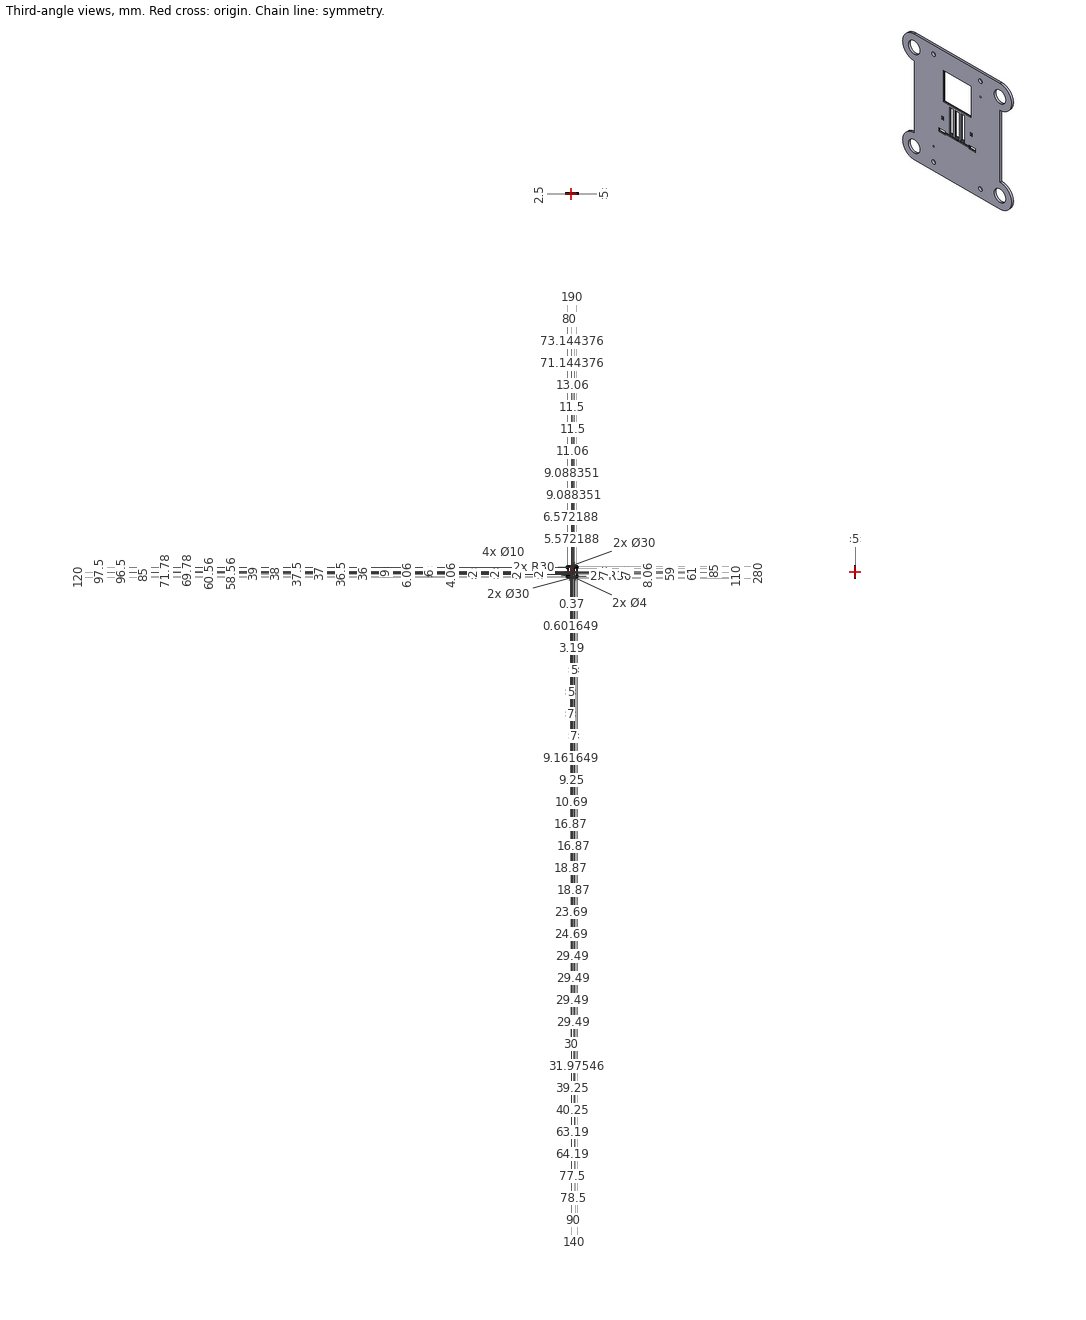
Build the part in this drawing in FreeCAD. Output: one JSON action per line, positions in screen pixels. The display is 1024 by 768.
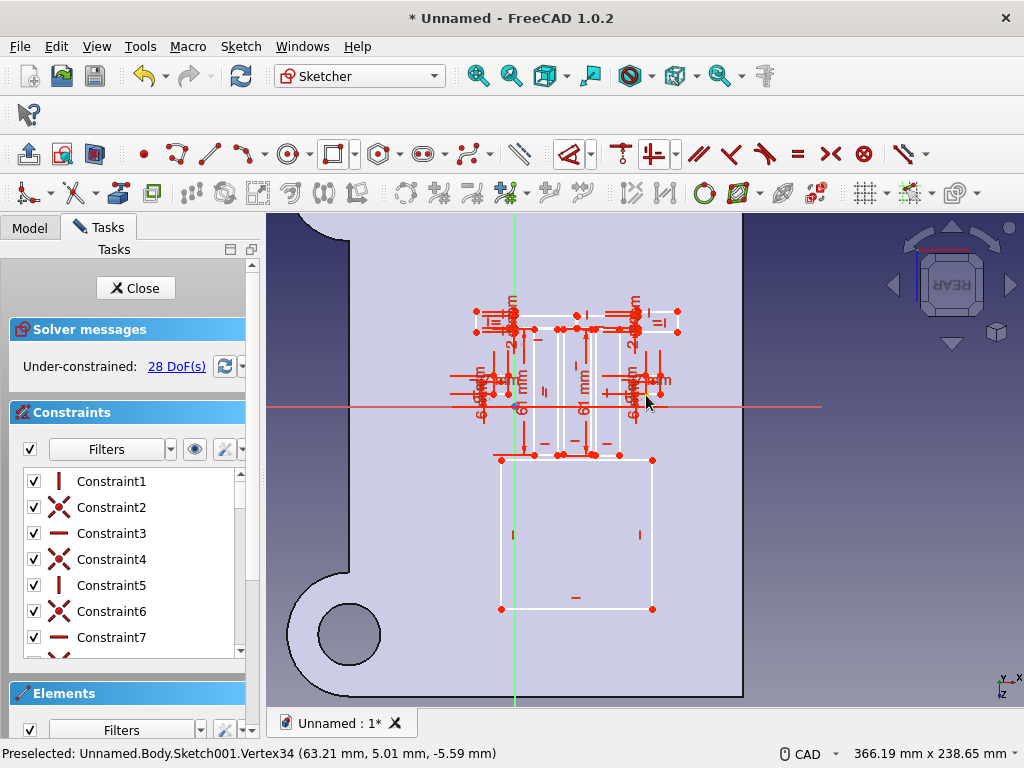
{"action": "scroll", "coordinate": [516, 332], "scroll_direction": "up", "scroll_amount": 6}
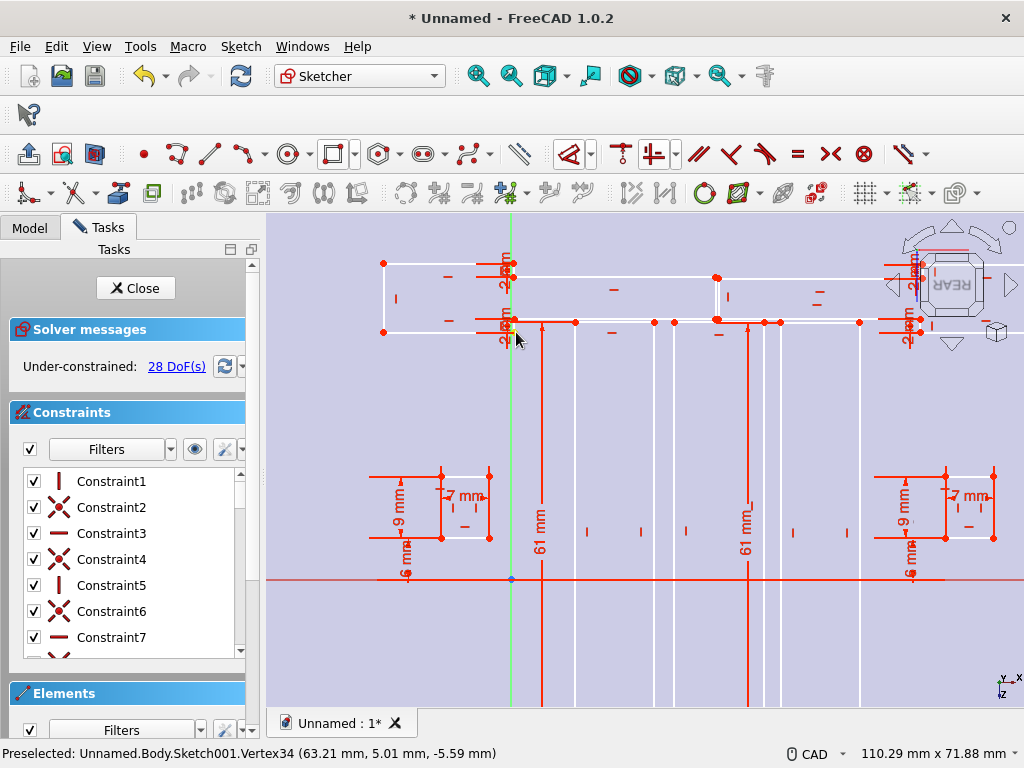
{"action": "left_click", "coordinate": [514, 333]}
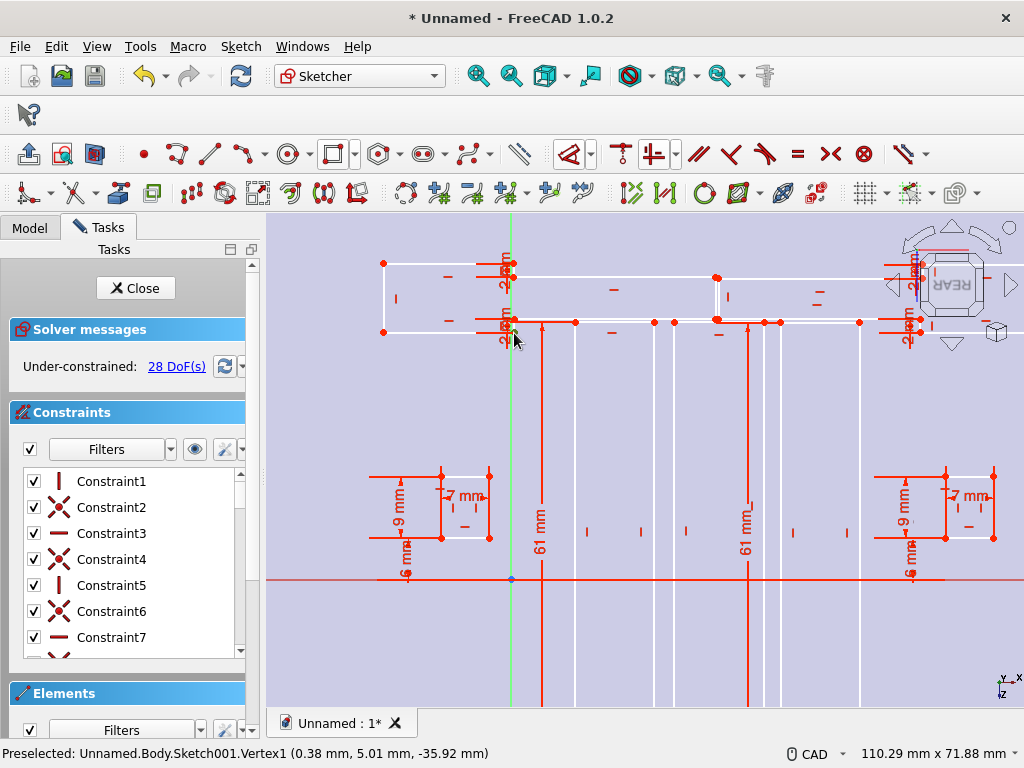
{"action": "left_click", "coordinate": [590, 154]}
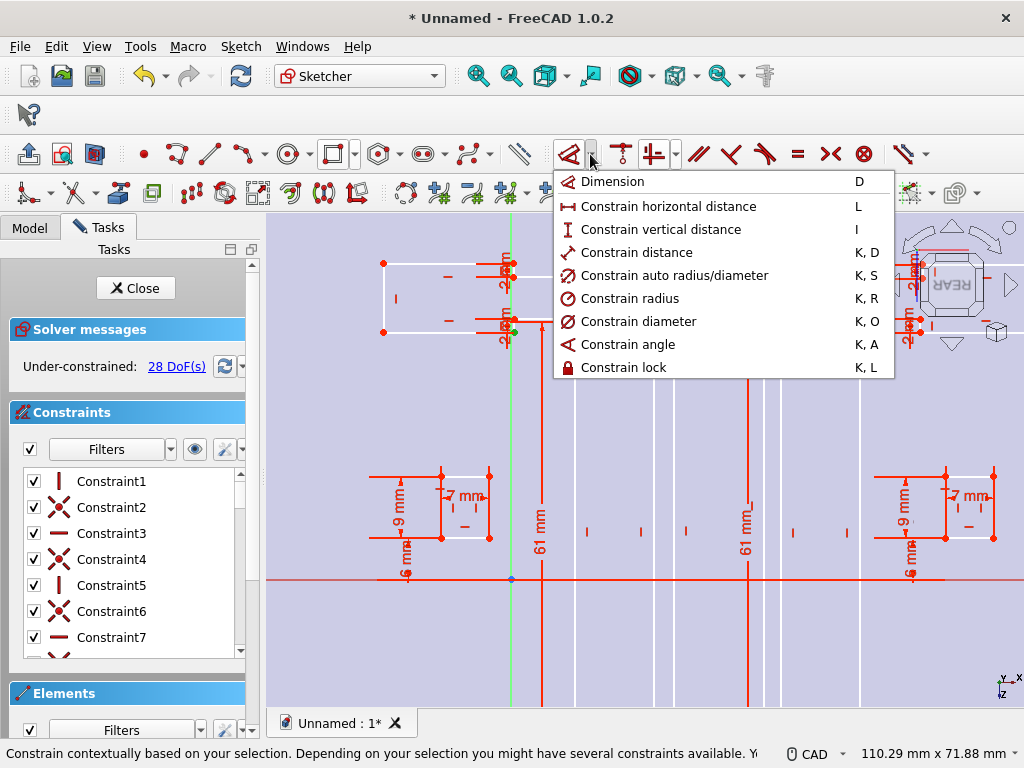
{"action": "left_click", "coordinate": [724, 230]}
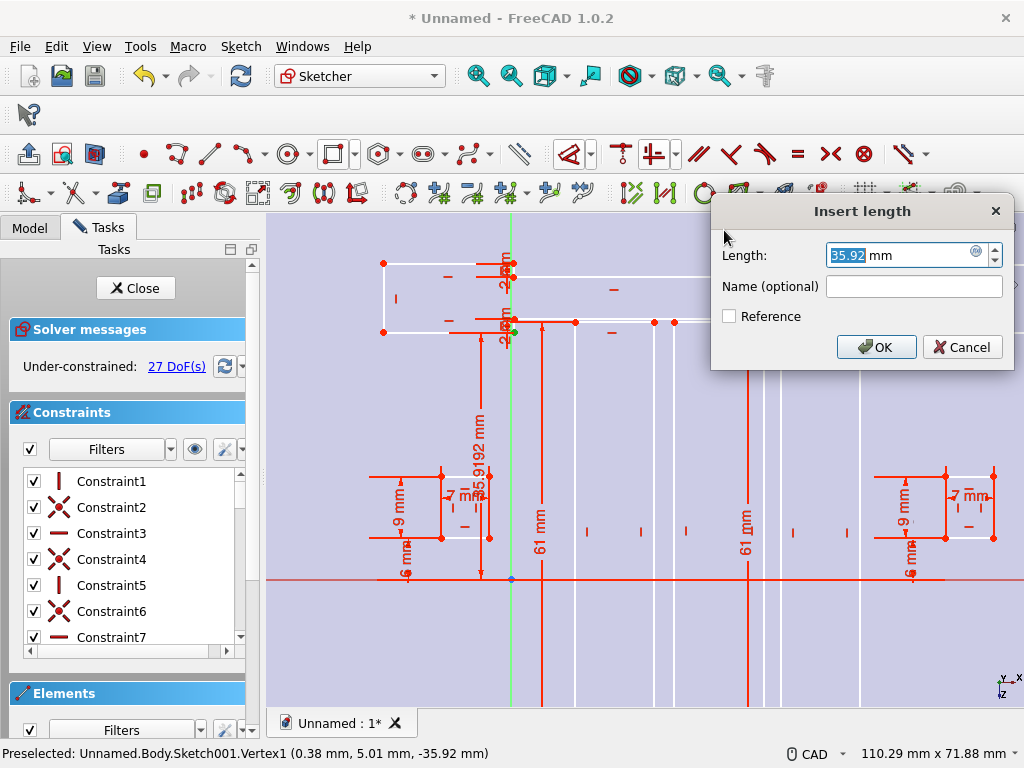
{"action": "type", "text": "36"}
{"action": "key", "text": "Return"}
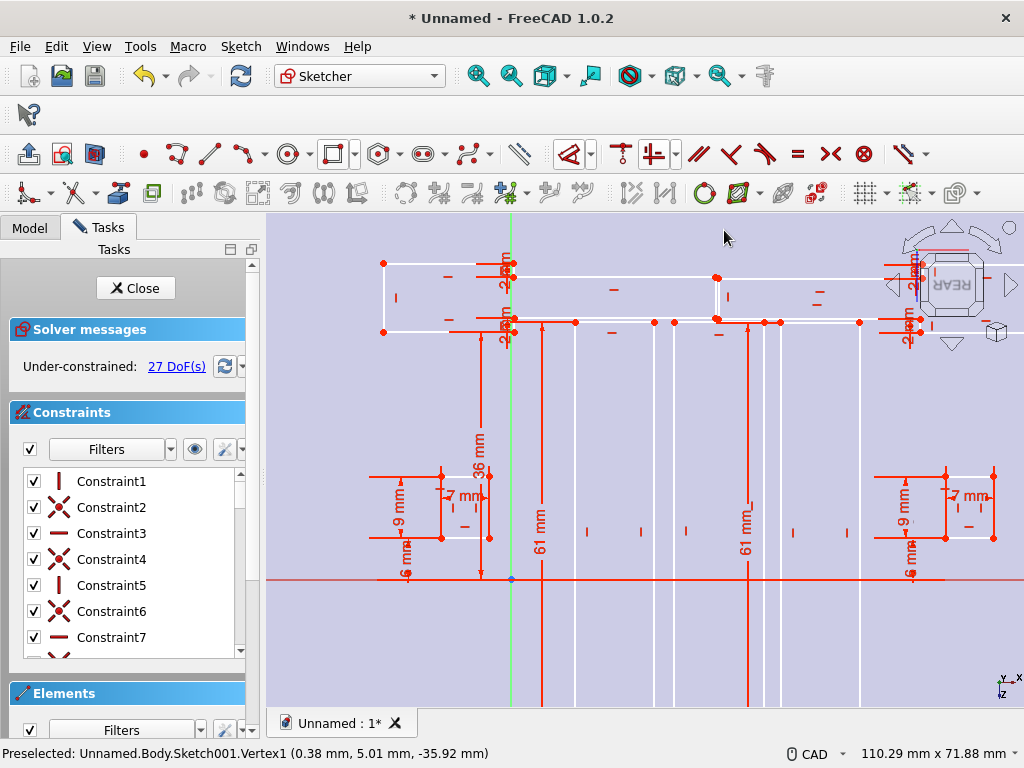
{"action": "scroll", "coordinate": [719, 319], "scroll_direction": "up", "scroll_amount": 7}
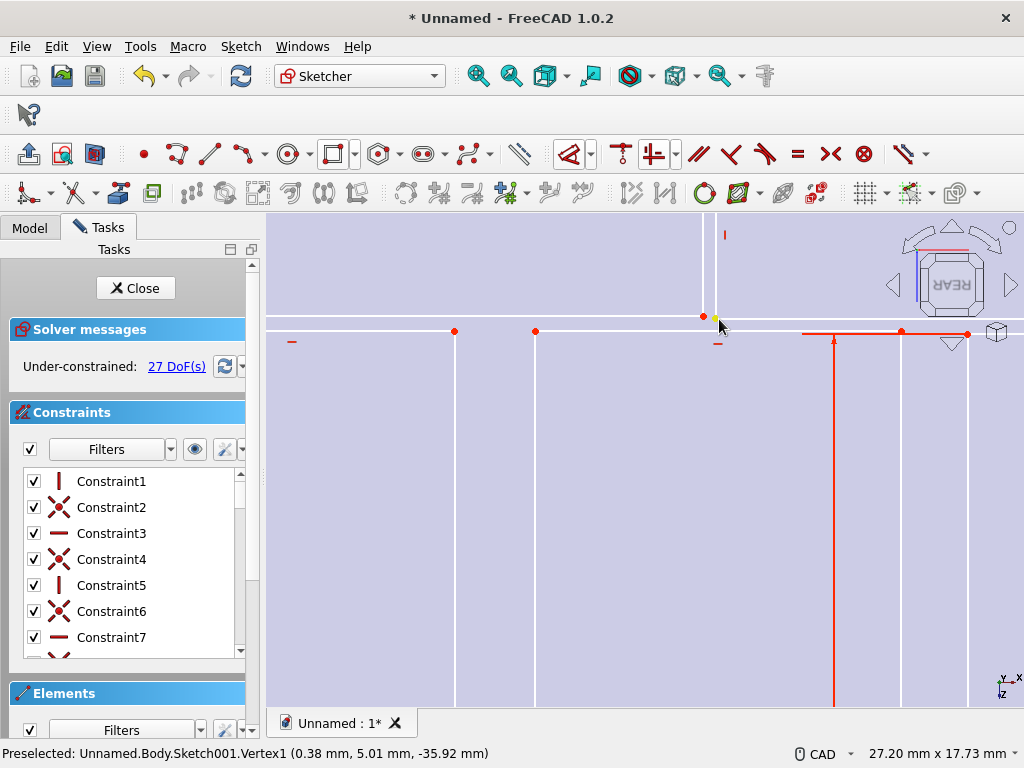
{"action": "left_click", "coordinate": [716, 319]}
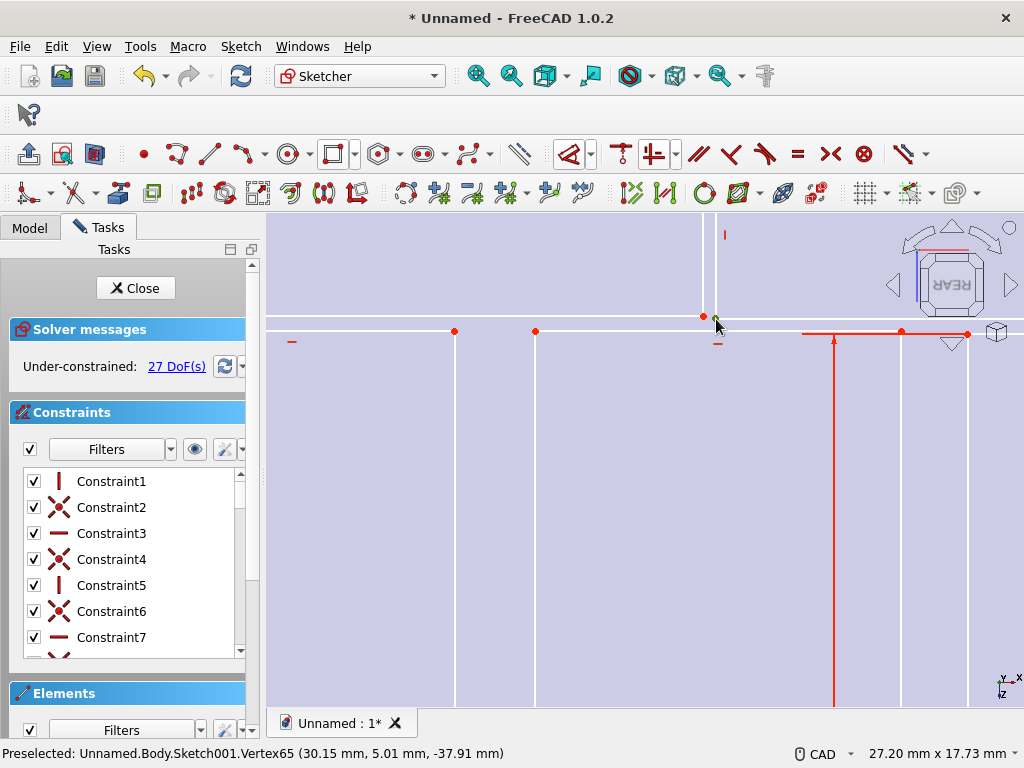
{"action": "left_click", "coordinate": [590, 154]}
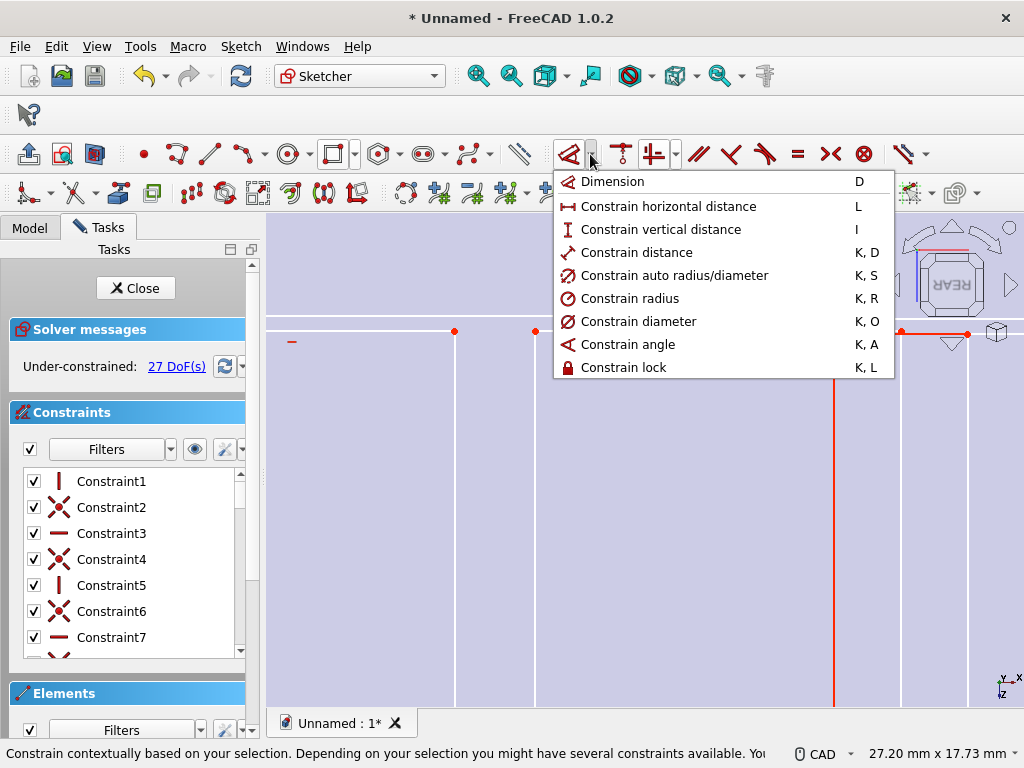
{"action": "left_click", "coordinate": [724, 230]}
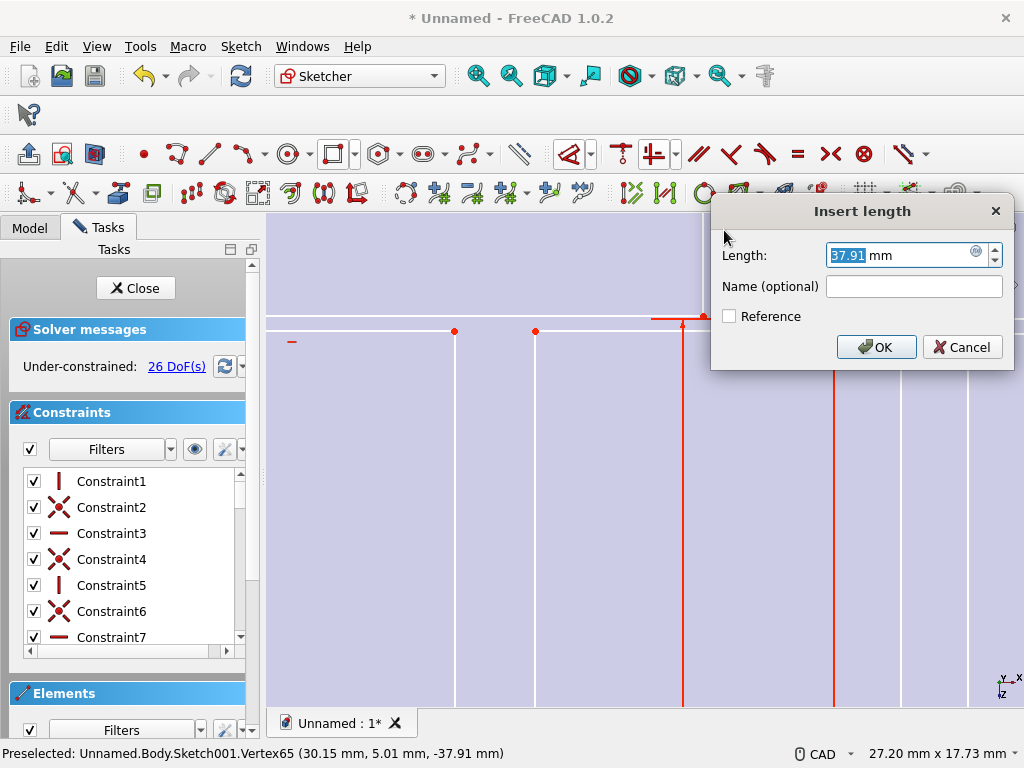
{"action": "type", "text": "38"}
{"action": "key", "text": "Return"}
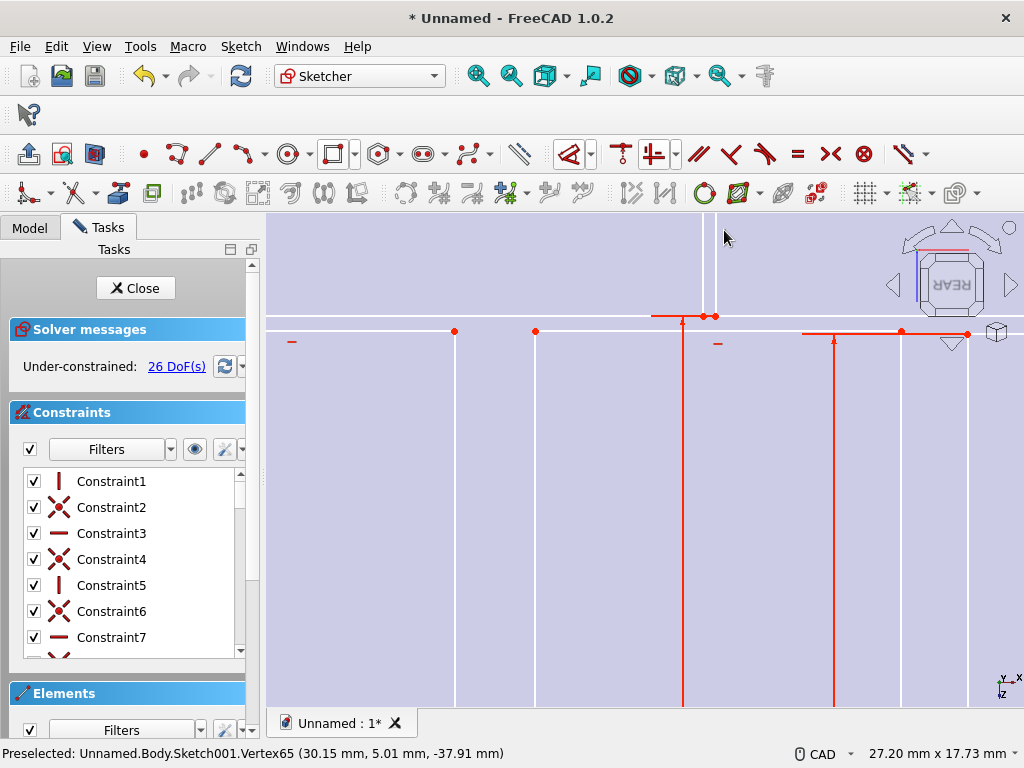
{"action": "left_click", "coordinate": [703, 266]}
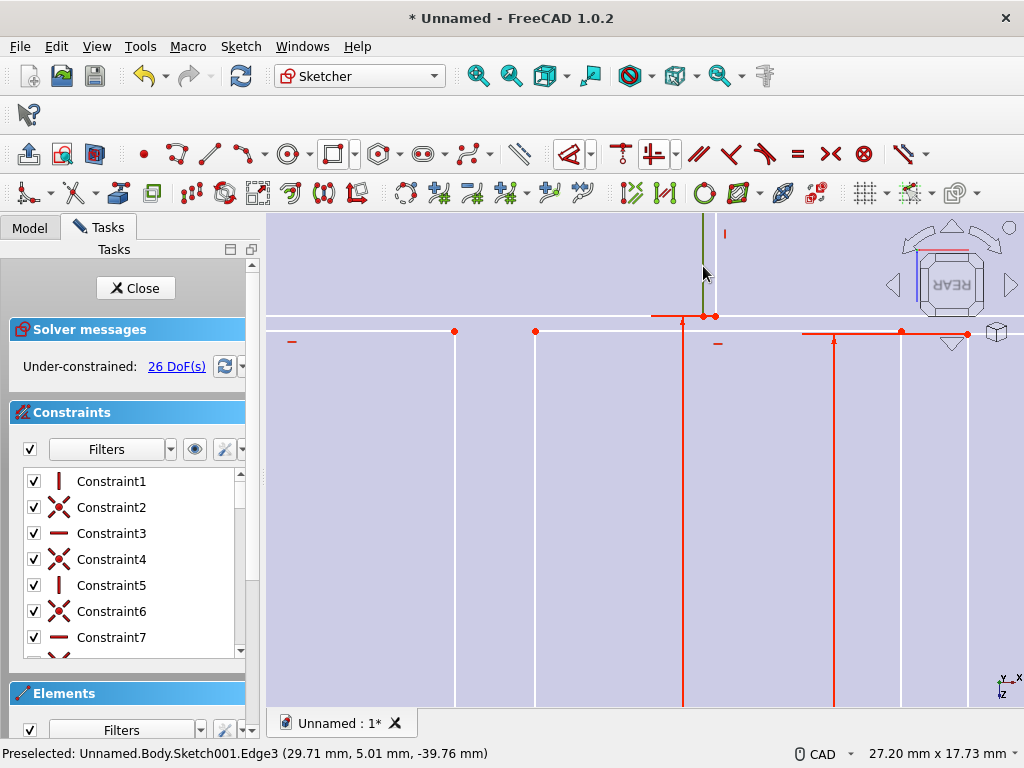
{"action": "key", "text": "i"}